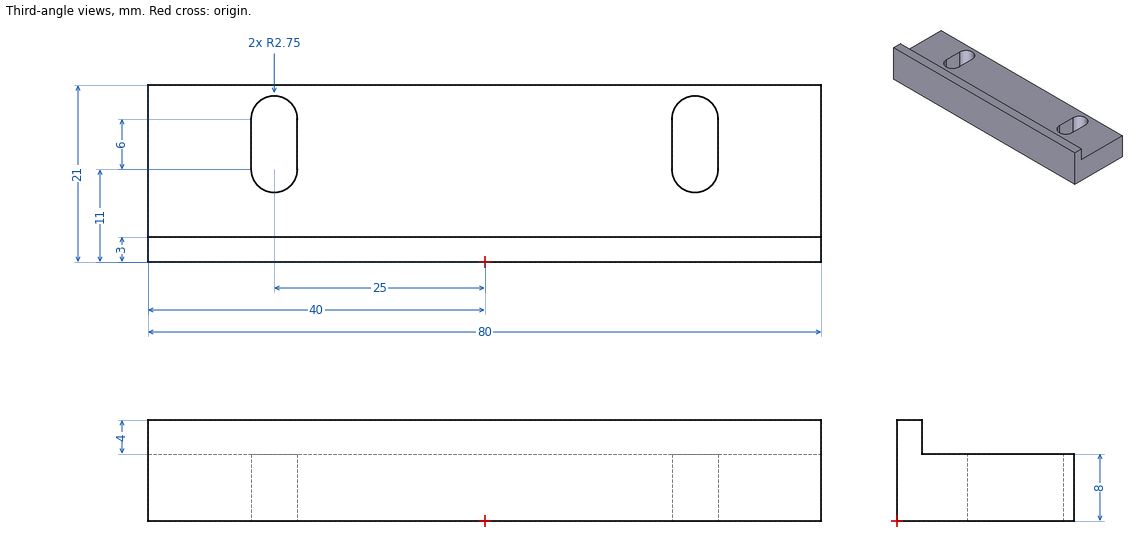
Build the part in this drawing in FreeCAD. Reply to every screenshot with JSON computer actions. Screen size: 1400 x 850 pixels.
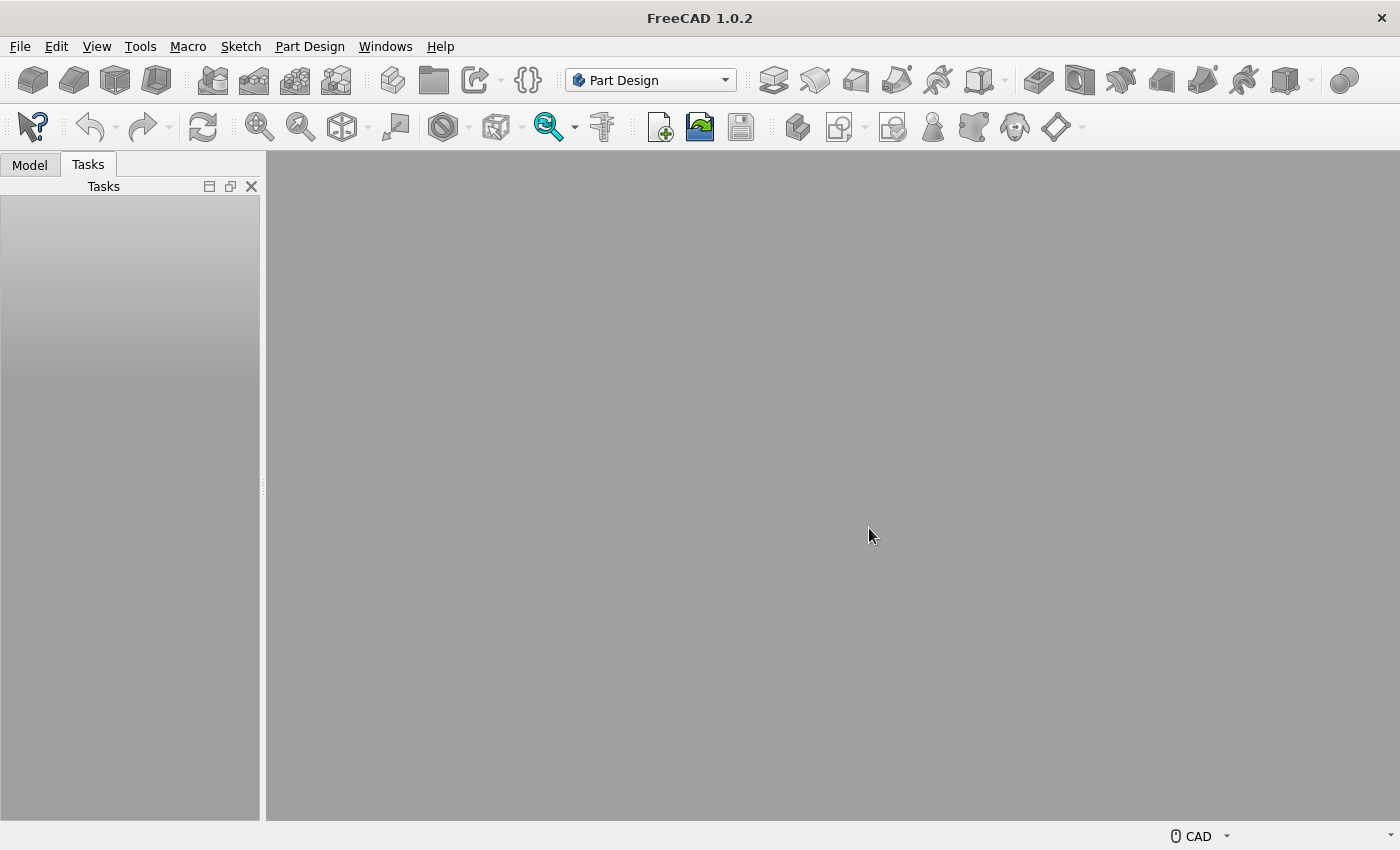
{"action": "key", "text": "ctrl+n"}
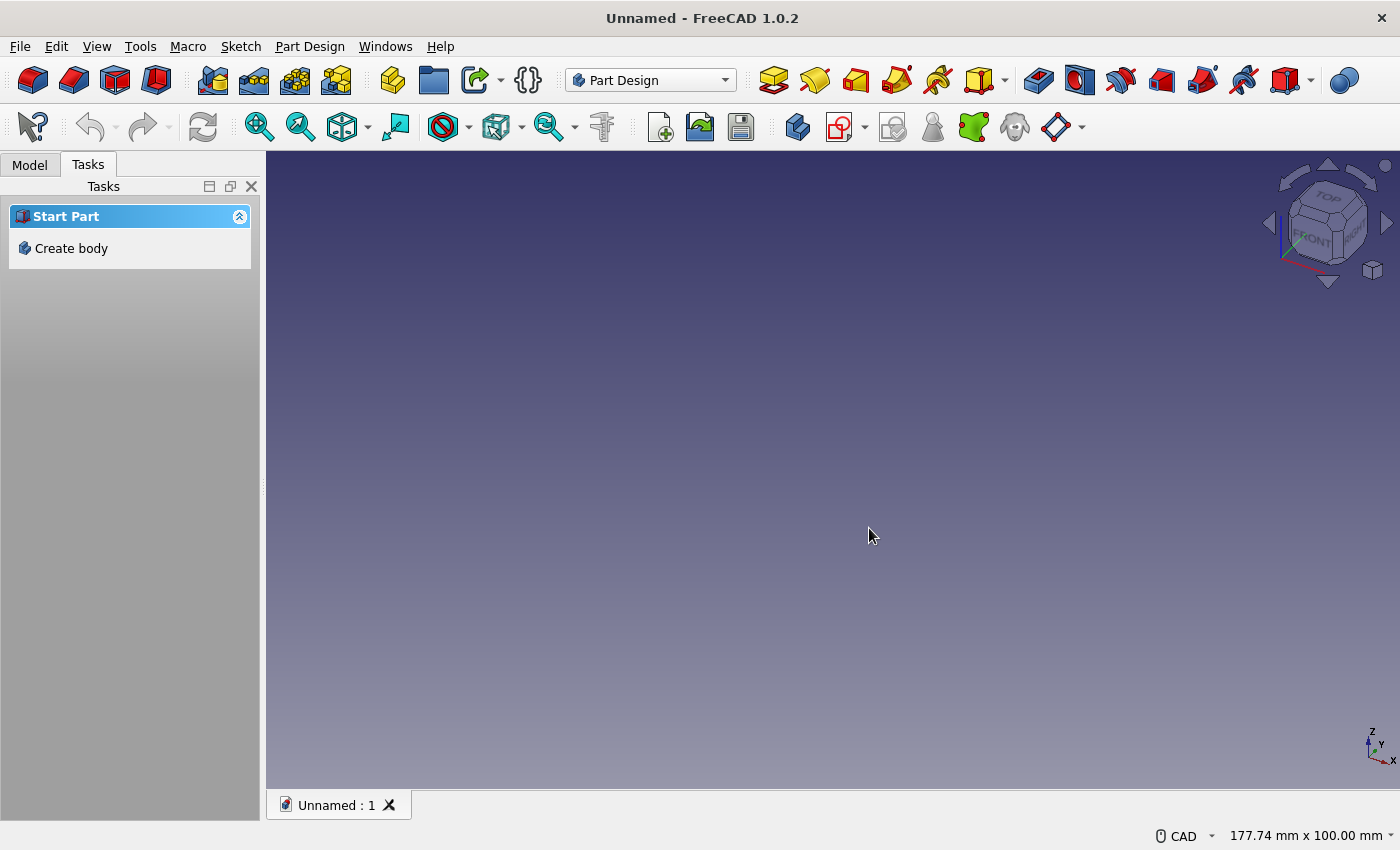
{"action": "left_click", "coordinate": [838, 128]}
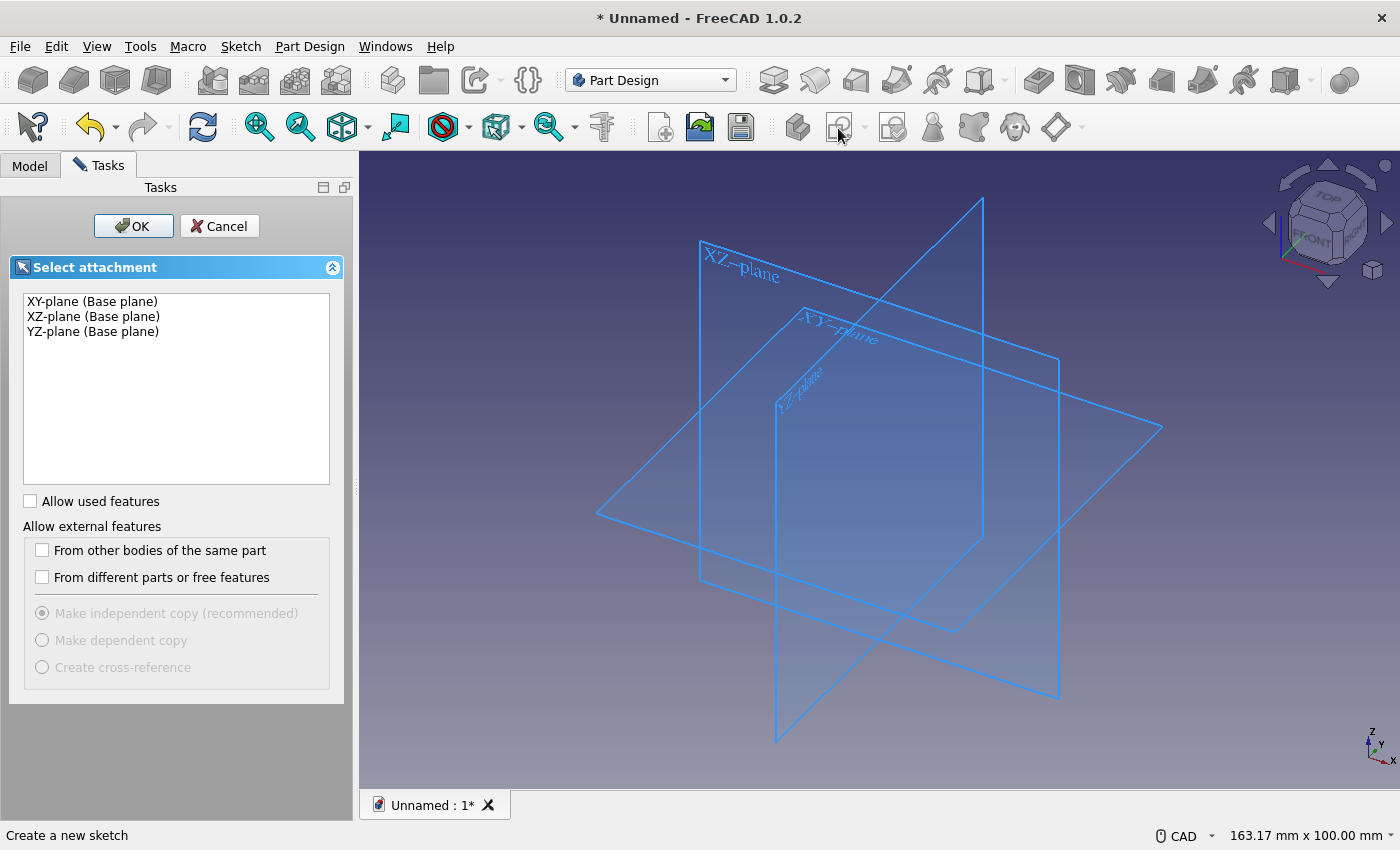
{"action": "left_click", "coordinate": [84, 302]}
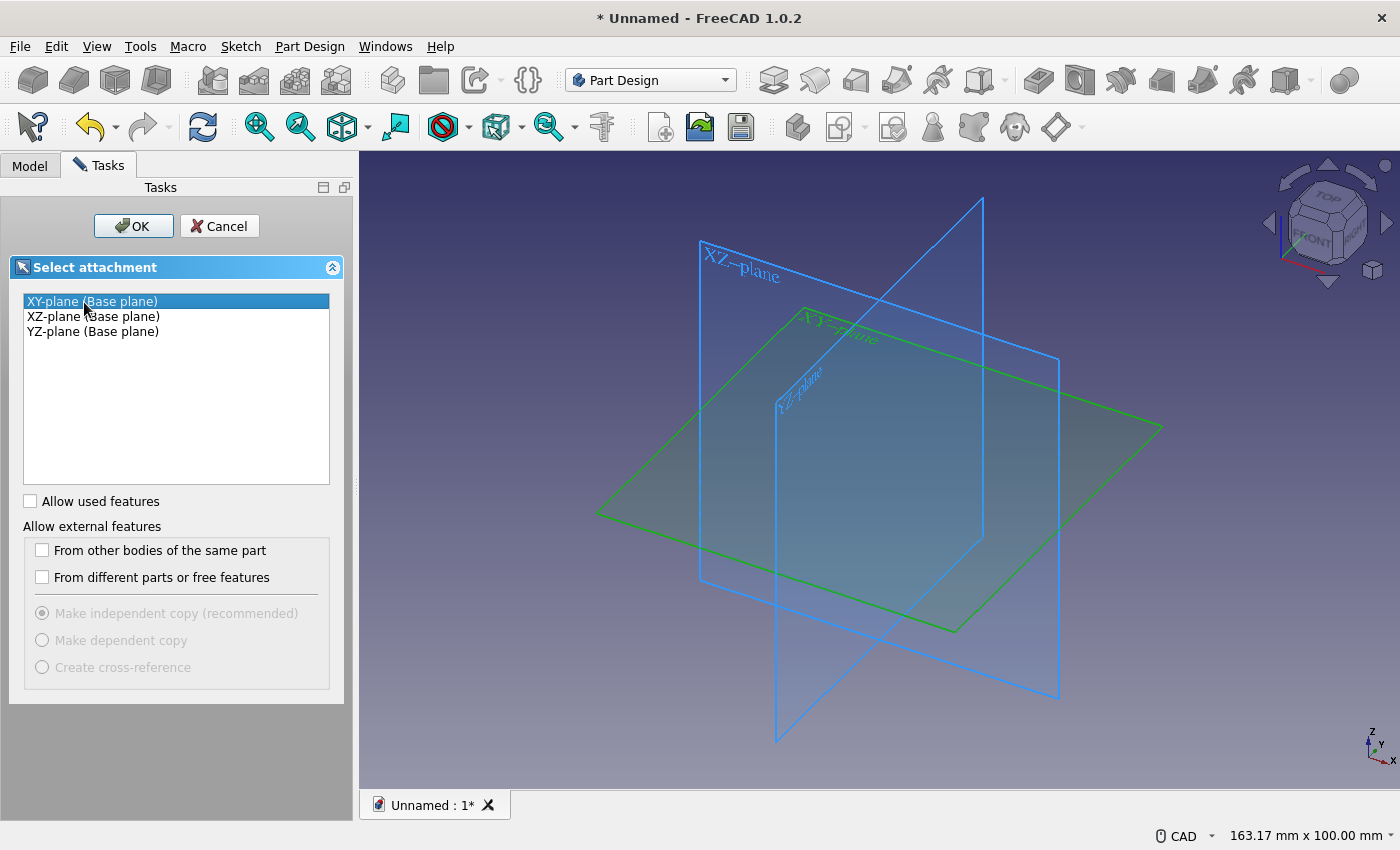
{"action": "left_click", "coordinate": [134, 226]}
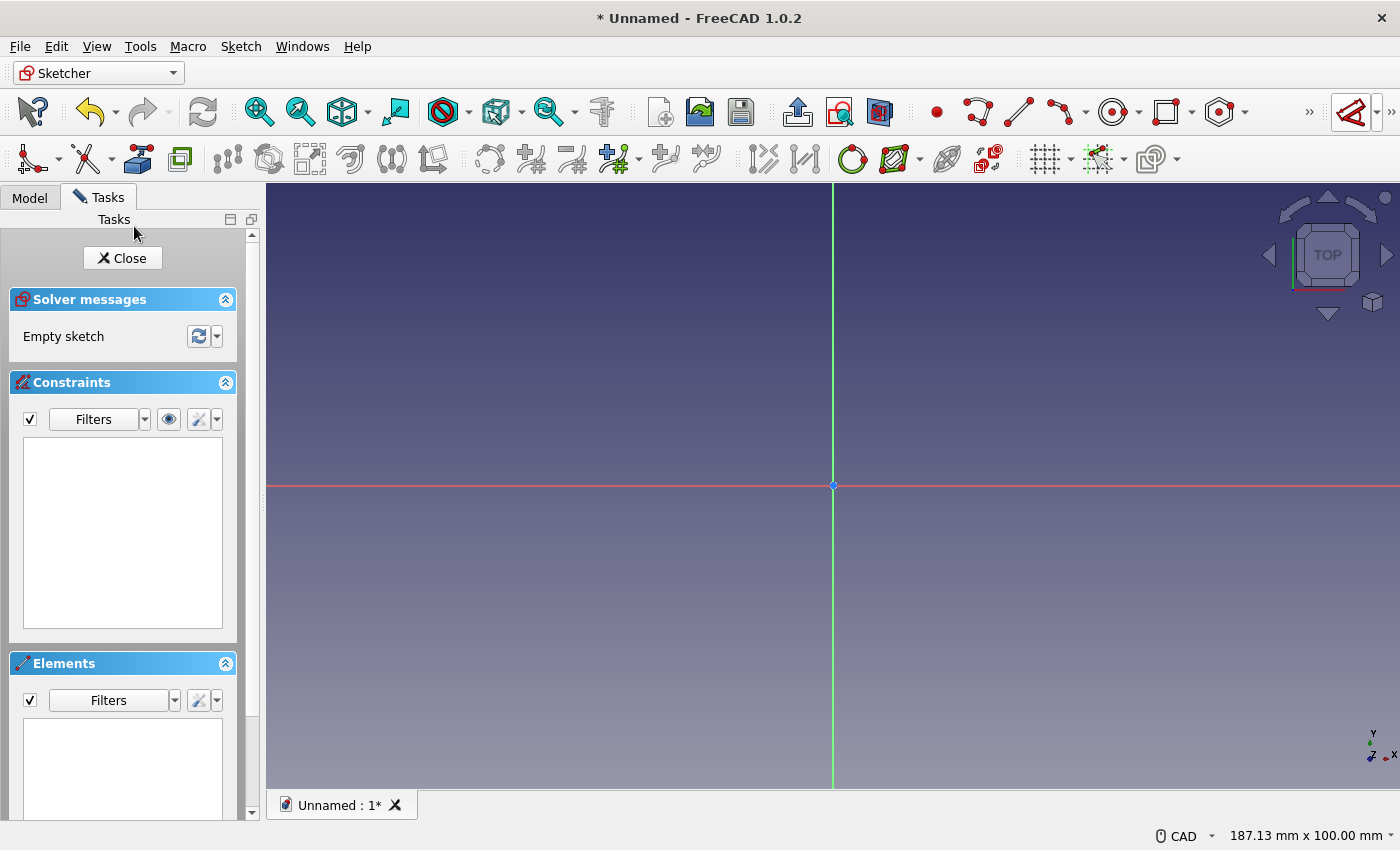
{"action": "scroll", "coordinate": [972, 293], "scroll_direction": "up", "scroll_amount": 2}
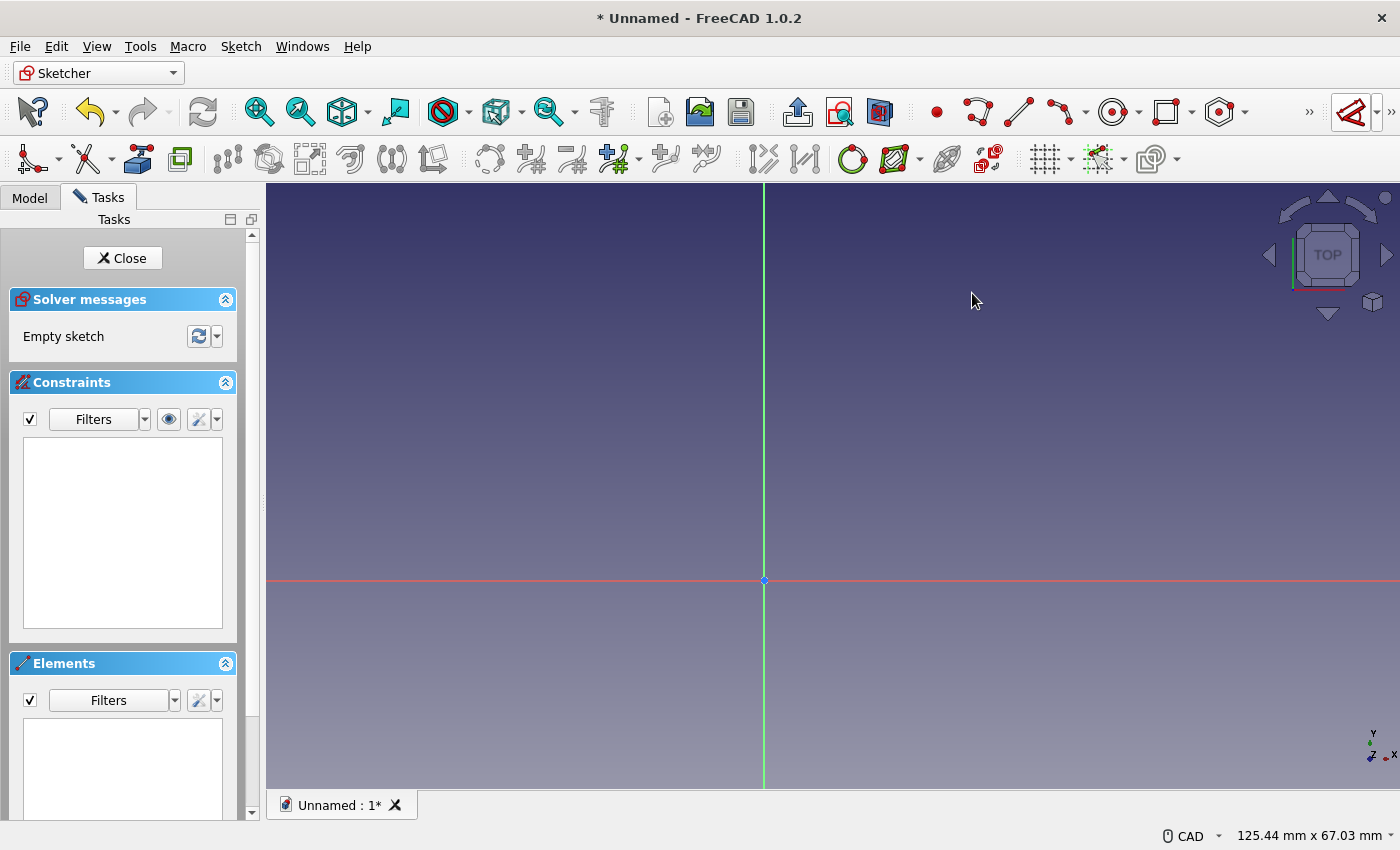
{"action": "key", "text": "g r"}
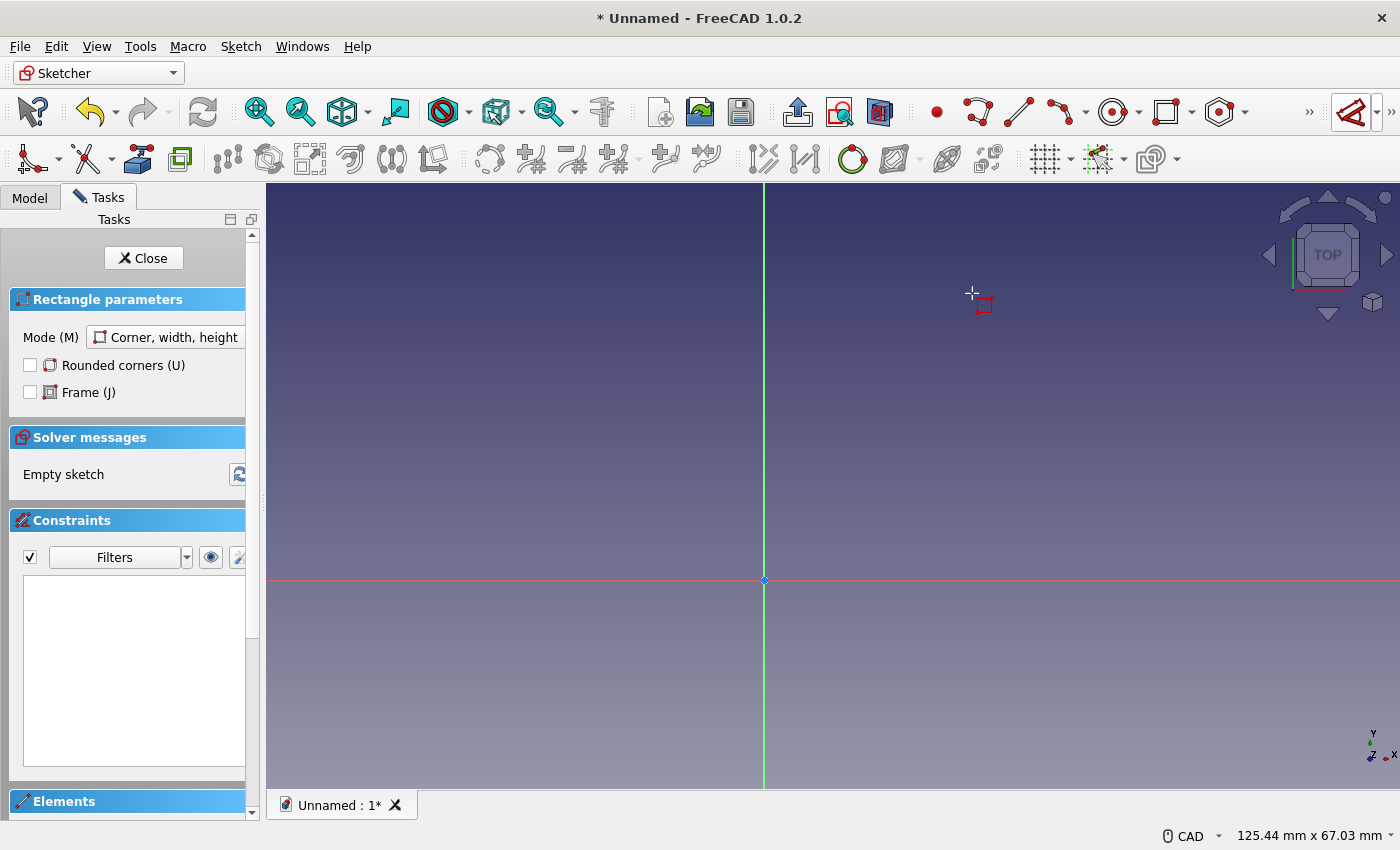
{"action": "left_click", "coordinate": [403, 391]}
{"action": "left_click", "coordinate": [1126, 581]}
{"action": "key", "text": "Escape"}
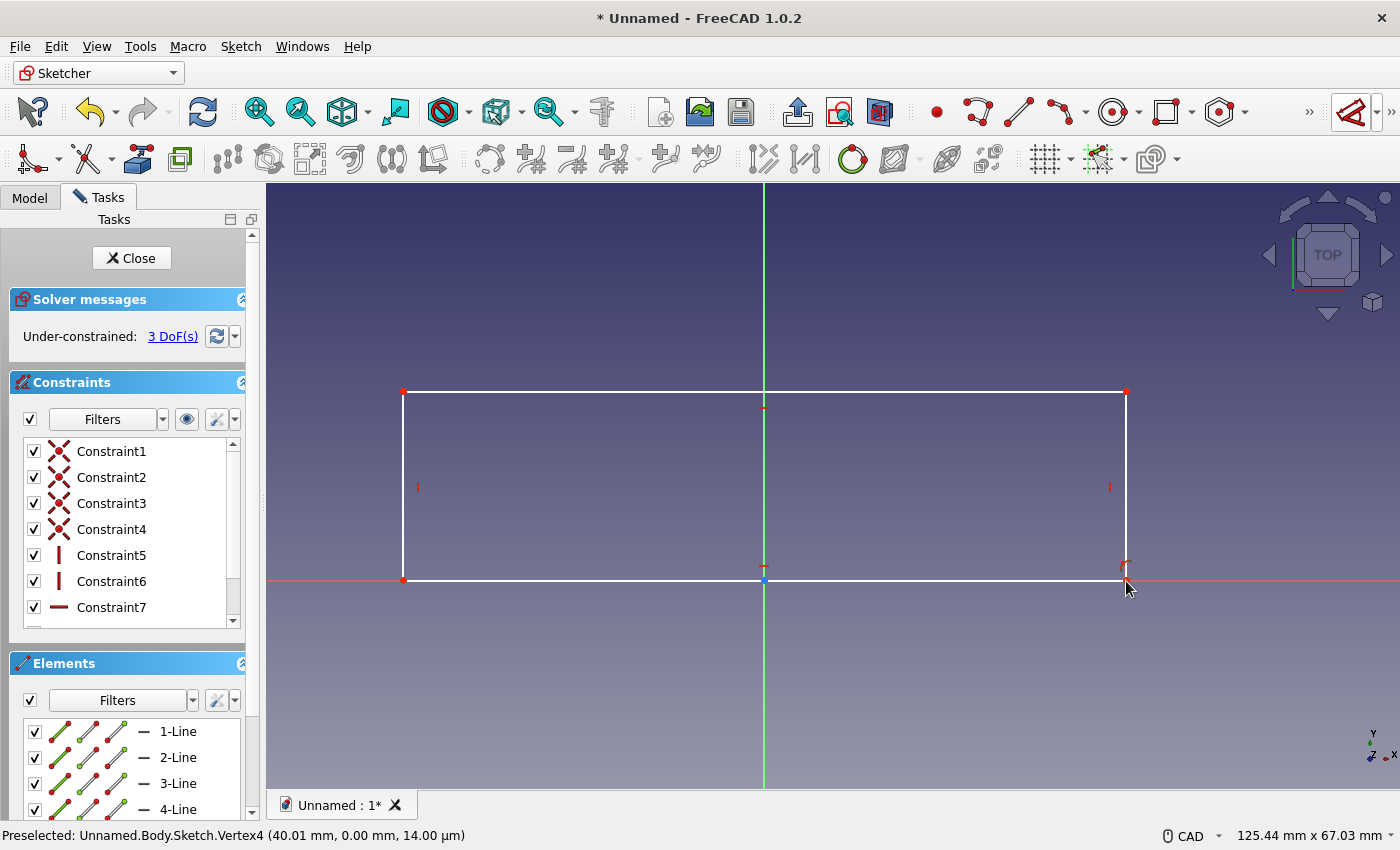
{"action": "key", "text": "d"}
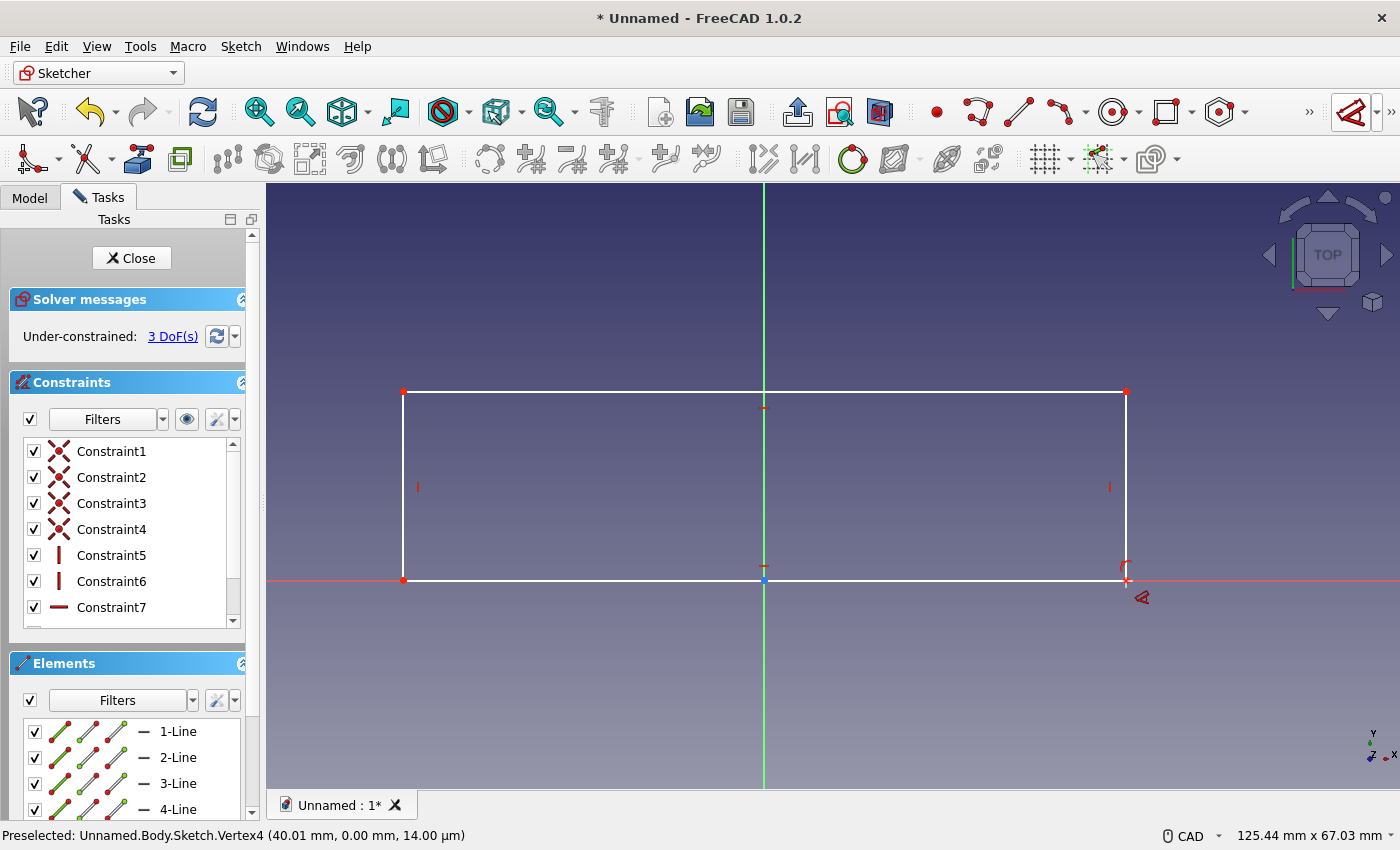
{"action": "left_click", "coordinate": [403, 449]}
{"action": "left_click", "coordinate": [369, 486]}